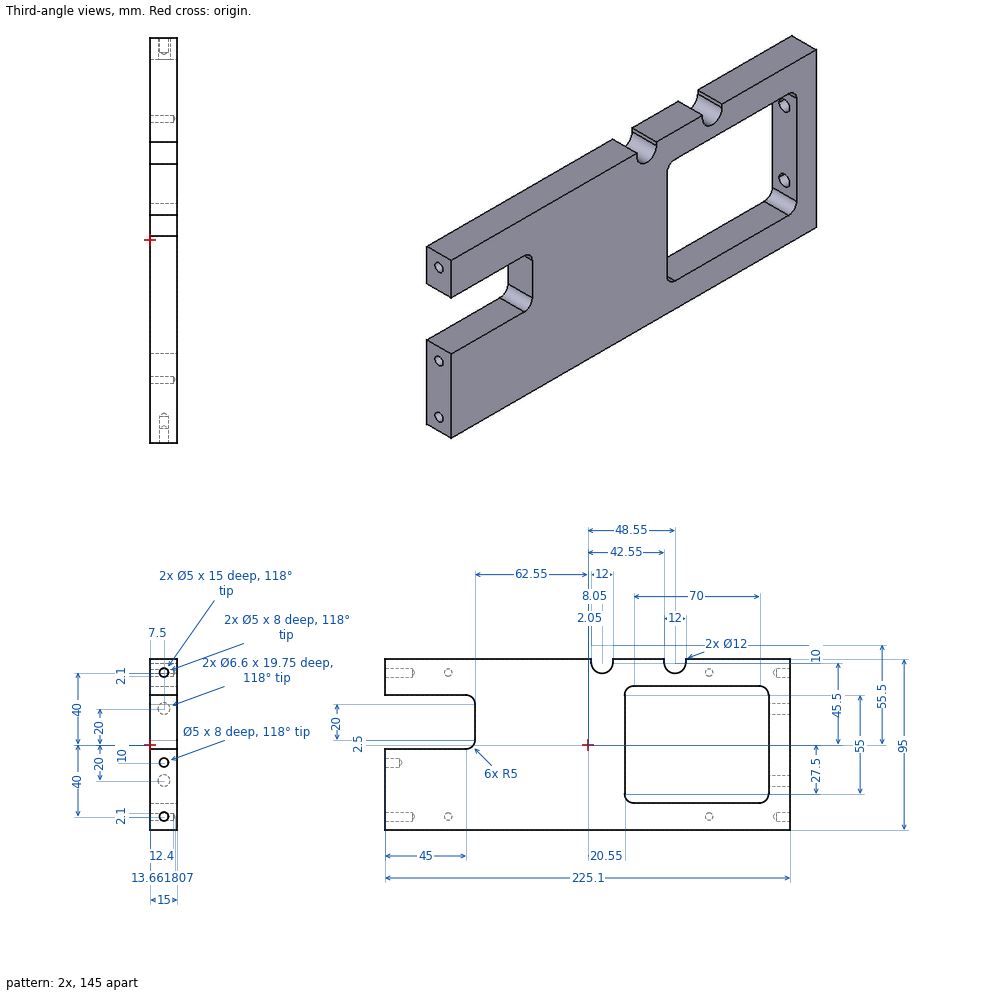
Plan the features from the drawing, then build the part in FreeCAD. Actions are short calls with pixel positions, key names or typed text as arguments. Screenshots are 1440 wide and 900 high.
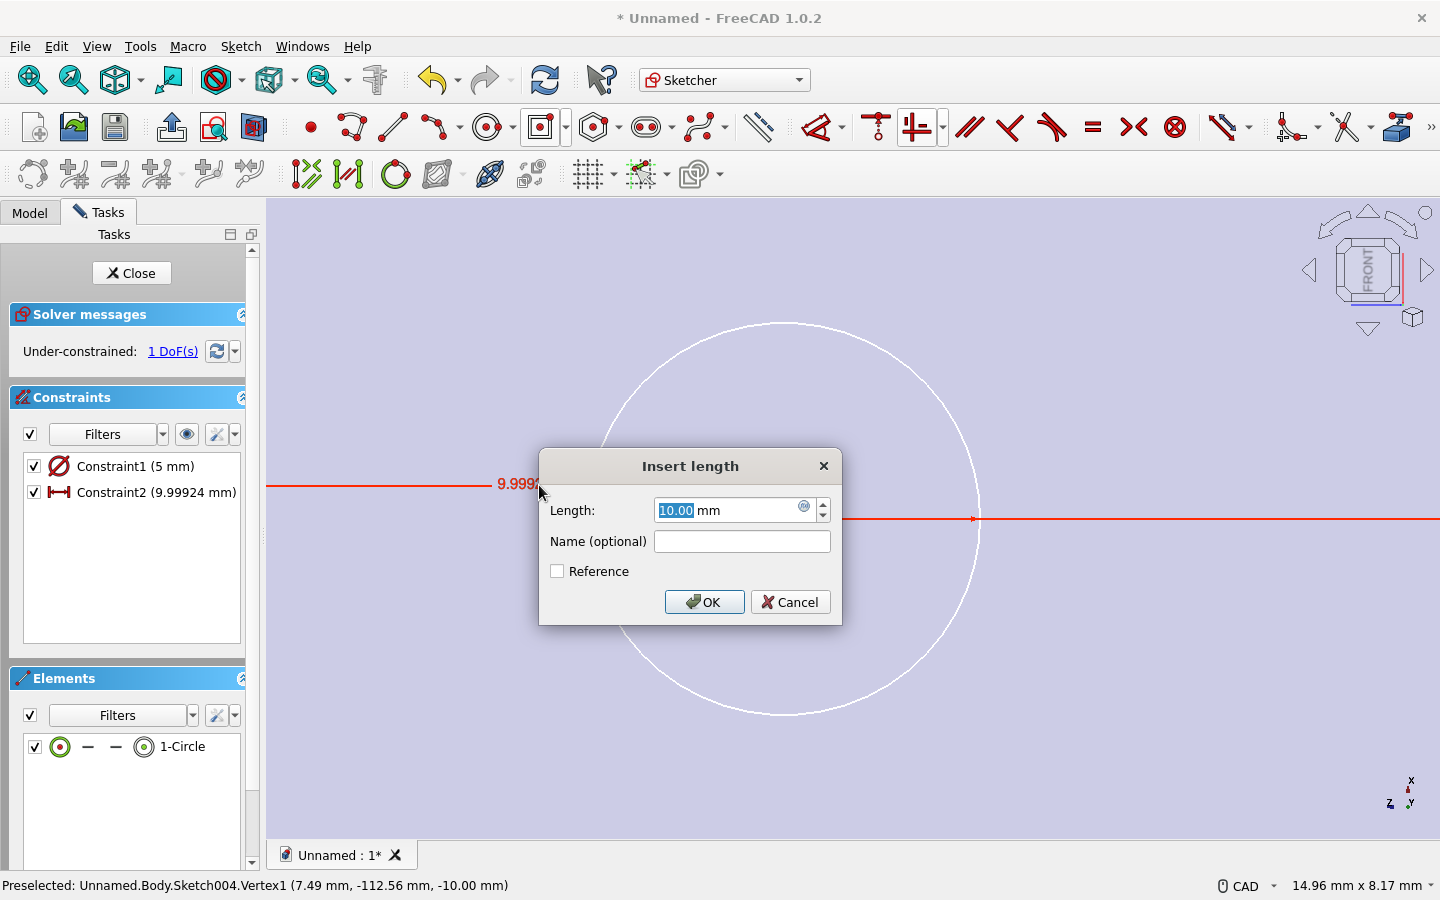
text(10)
key(Return)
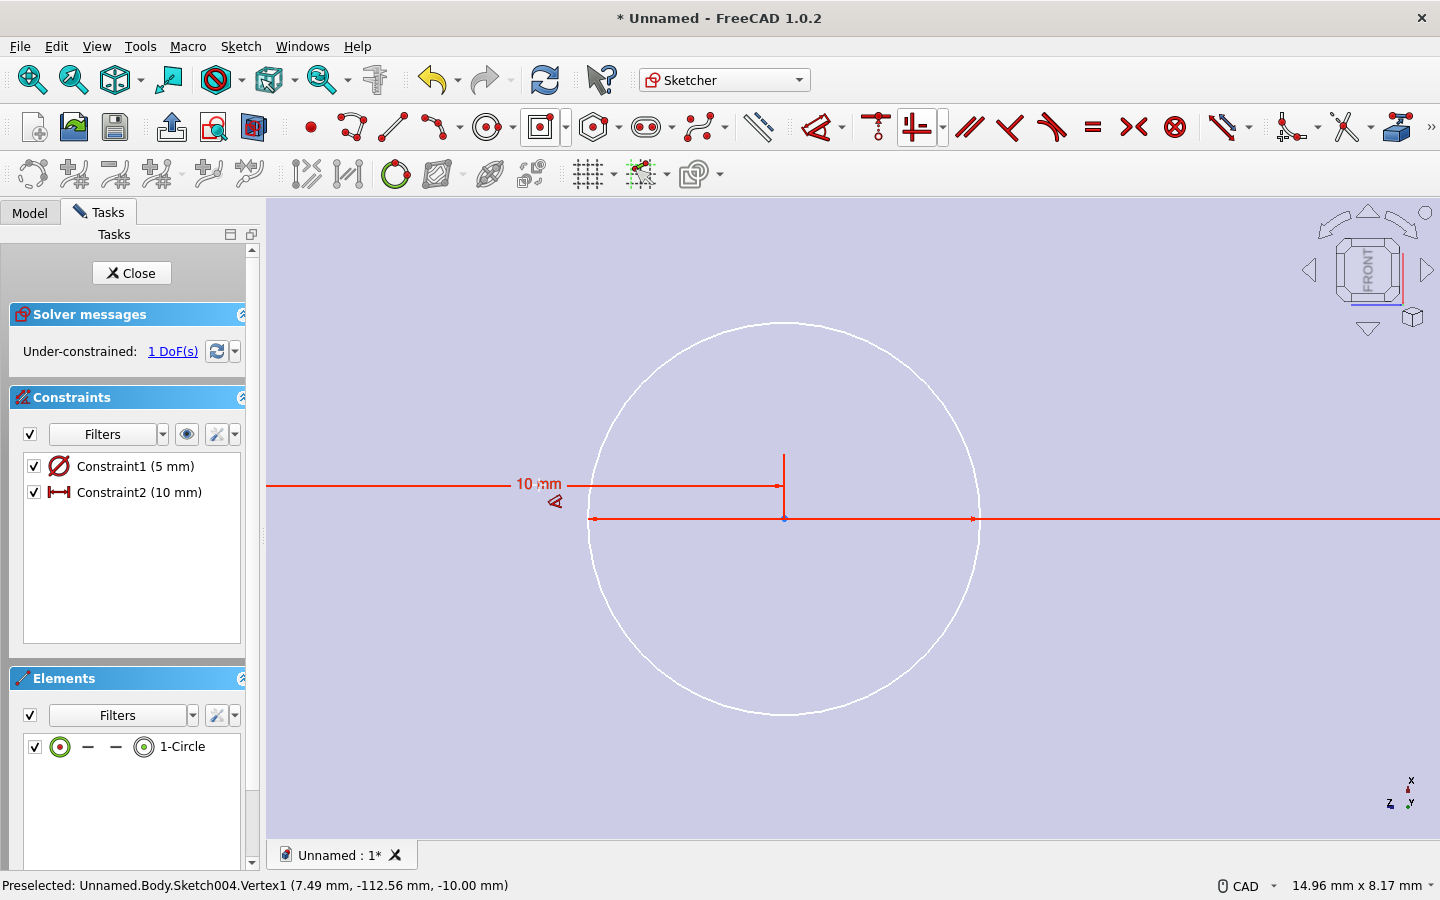
click(784, 519)
click(818, 665)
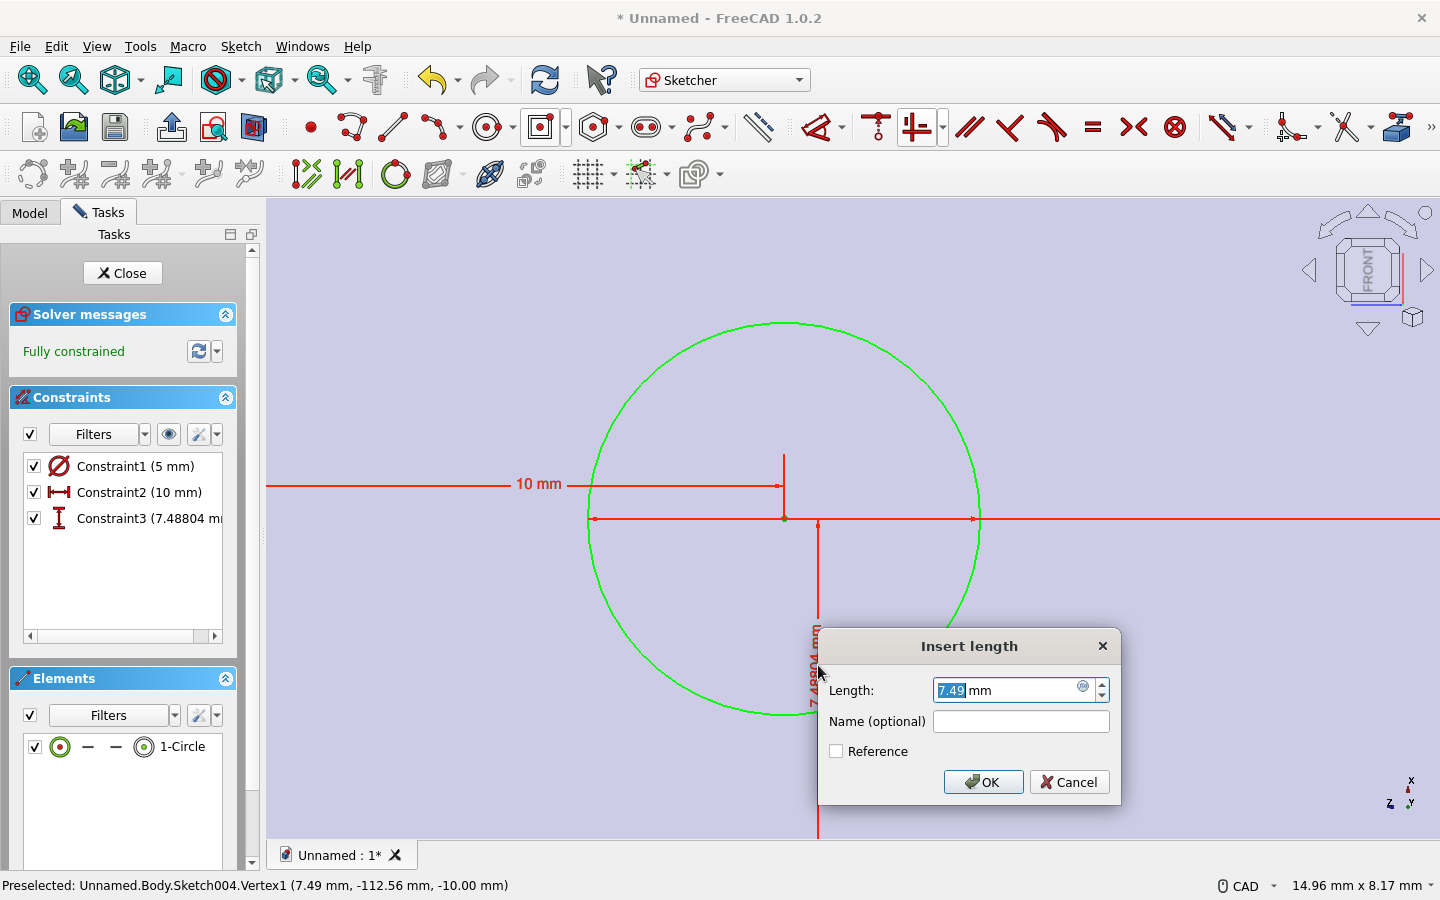
text(7.5)
key(Return)
key(Escape)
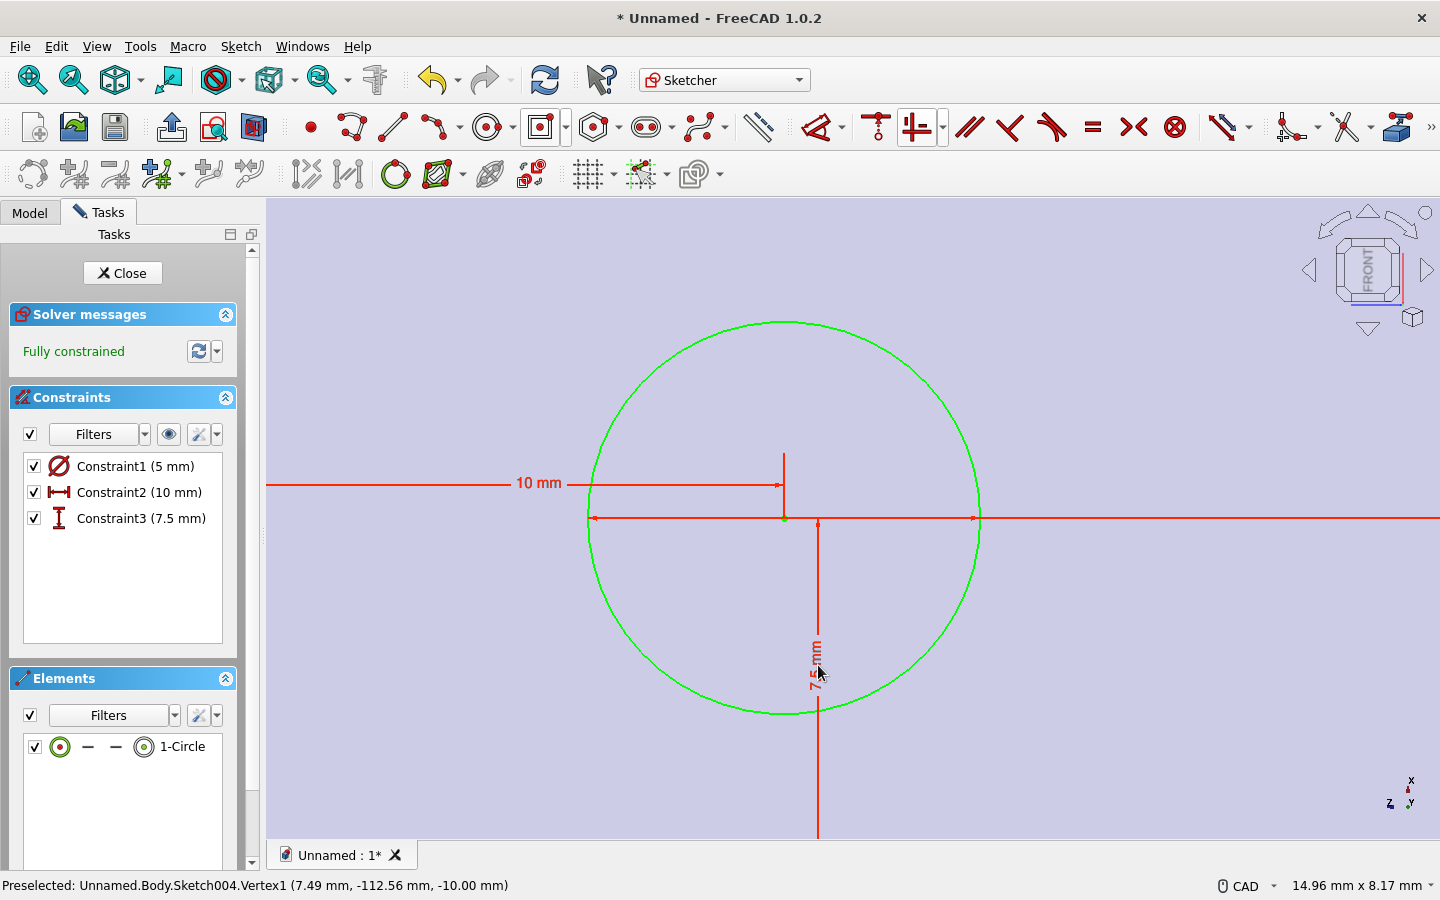
click(123, 273)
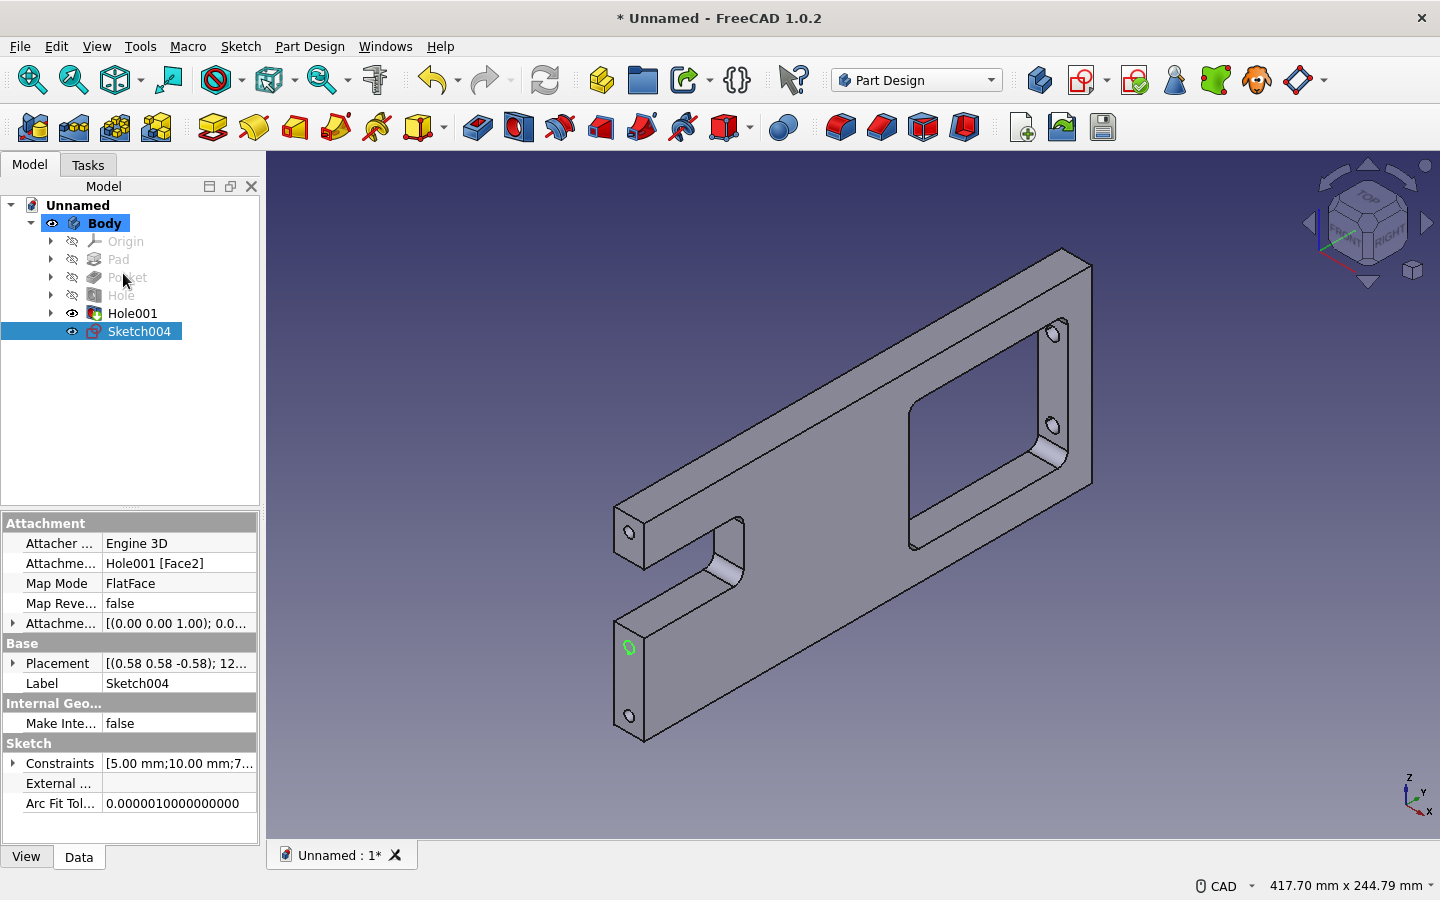
click(519, 128)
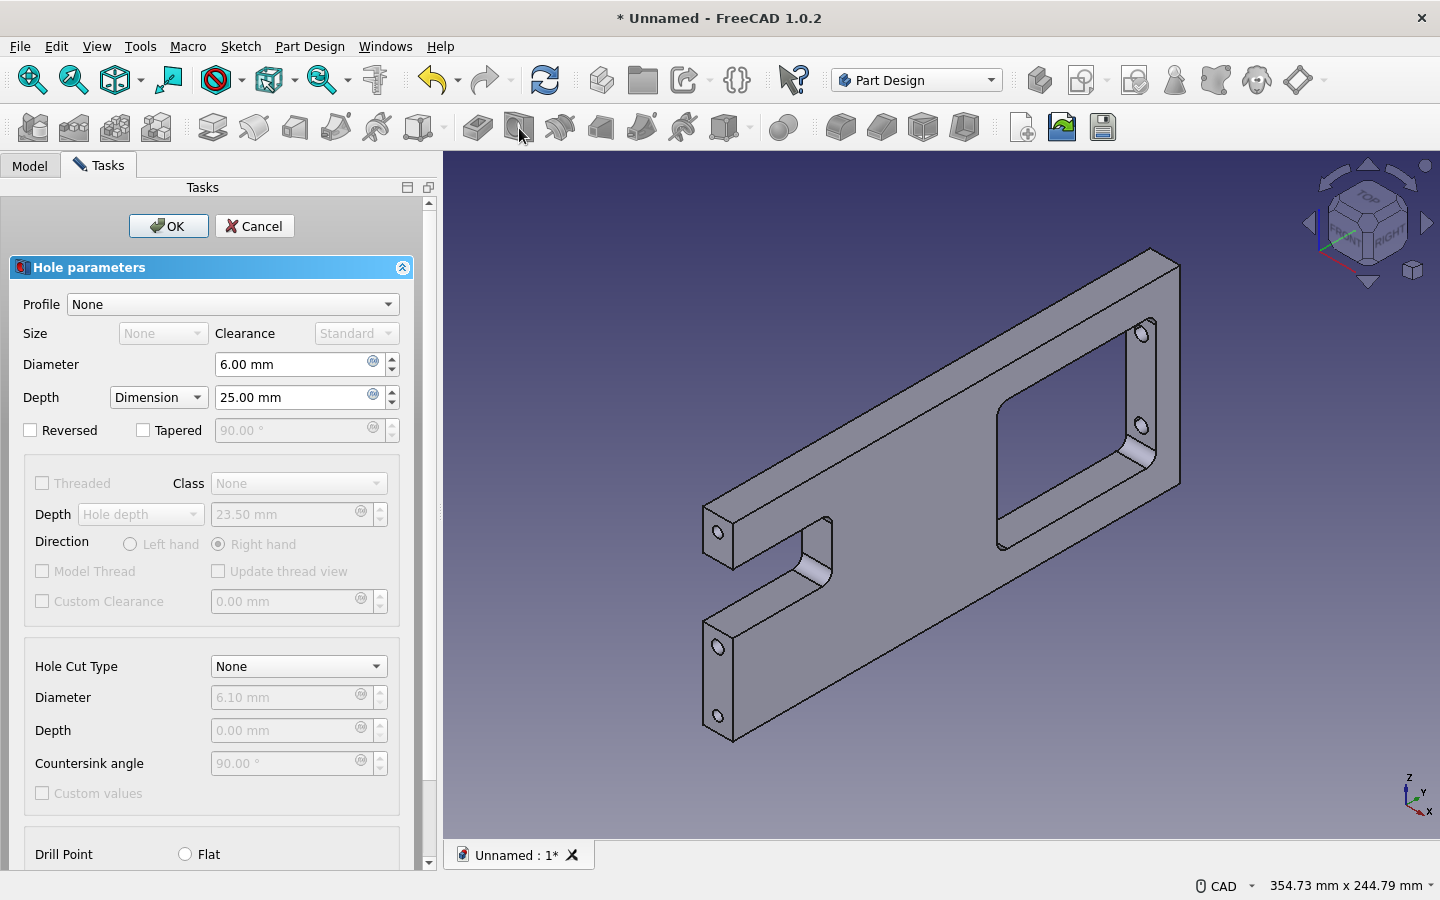
triple_click(300, 364)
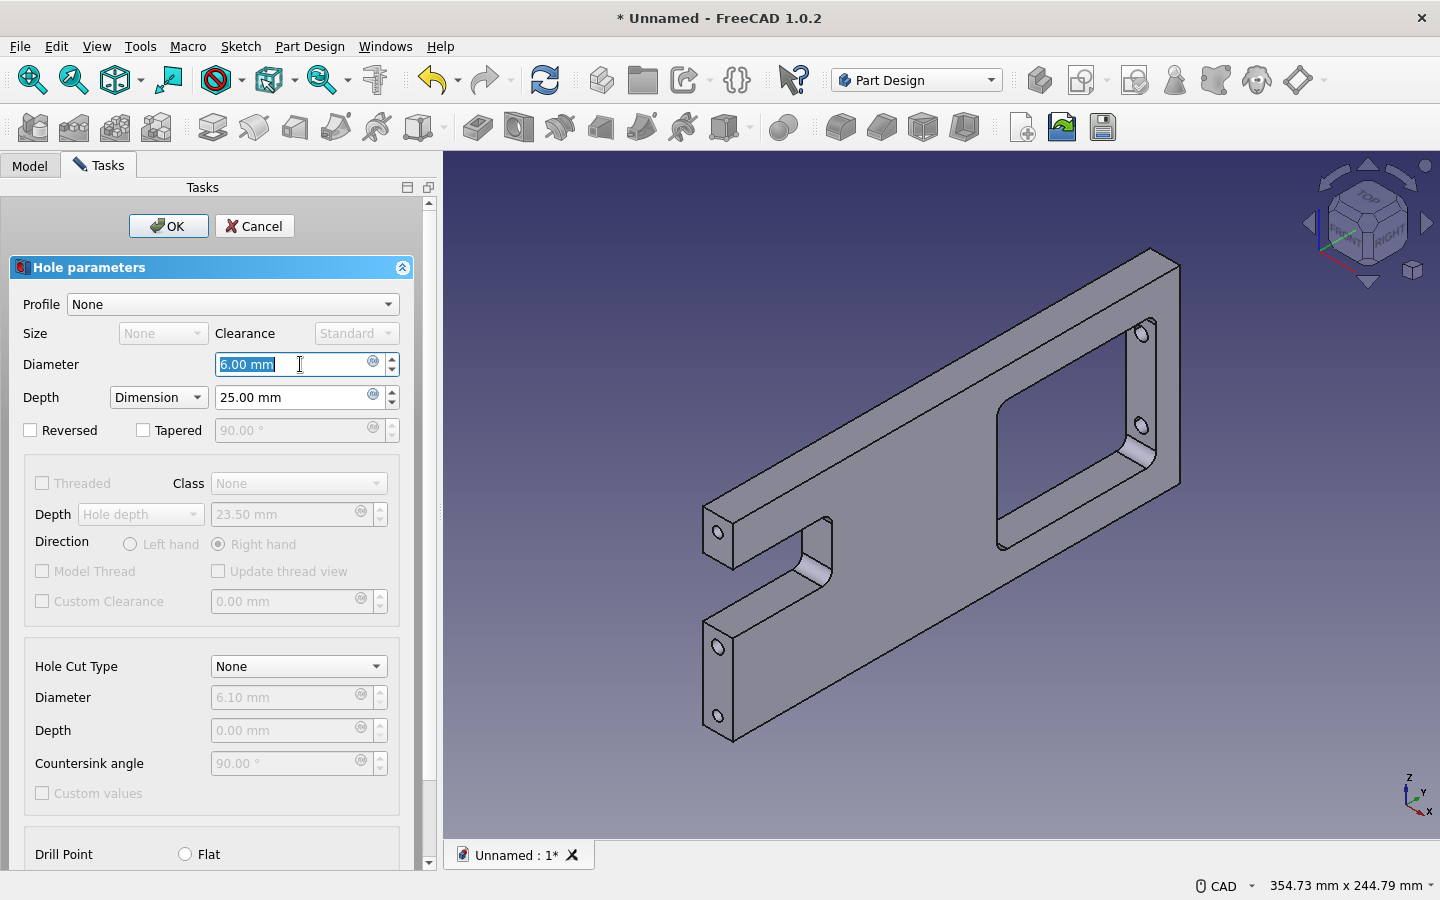
text(5)
key(Tab)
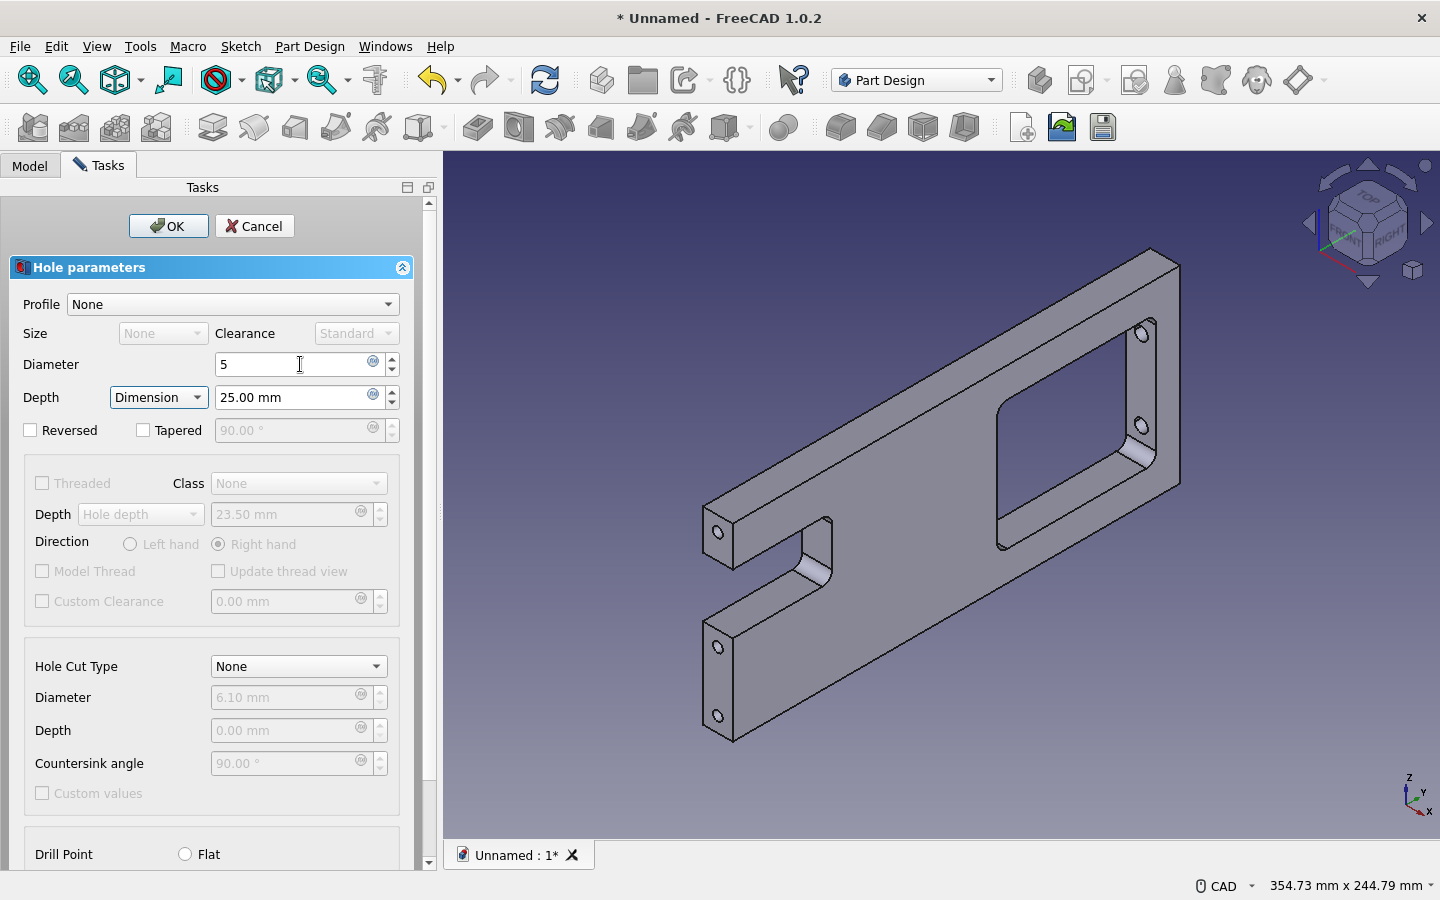
triple_click(300, 398)